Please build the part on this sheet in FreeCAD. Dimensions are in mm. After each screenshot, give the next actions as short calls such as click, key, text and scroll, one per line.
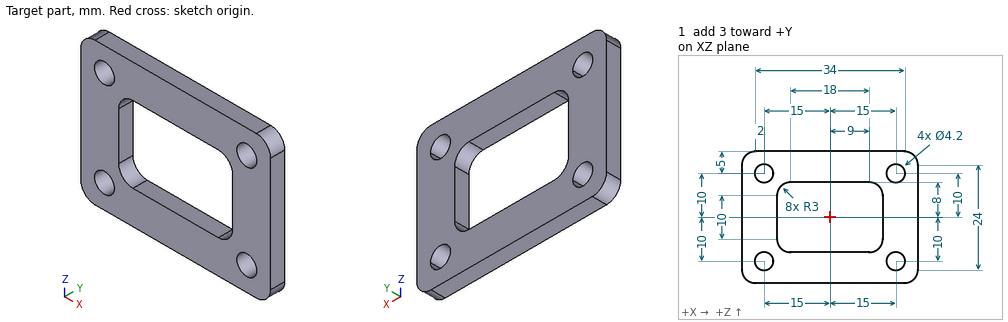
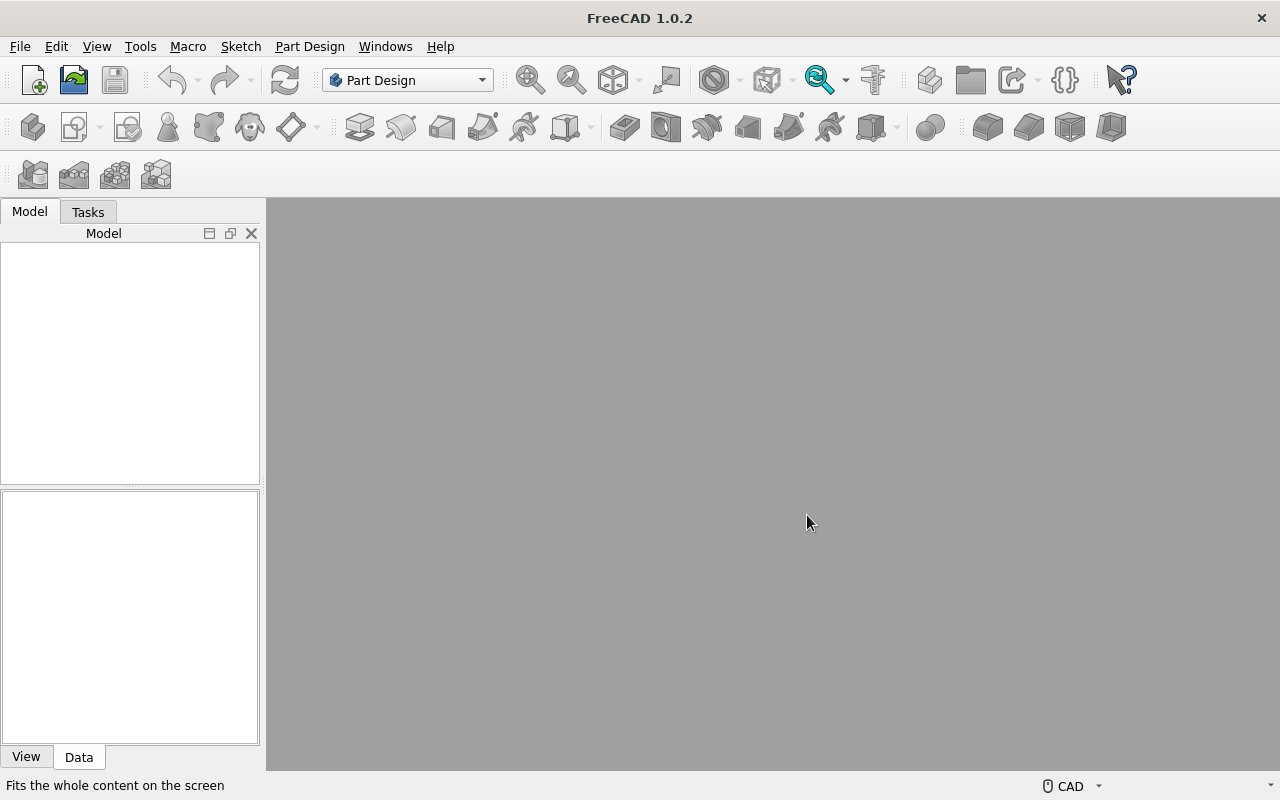
click(33, 80)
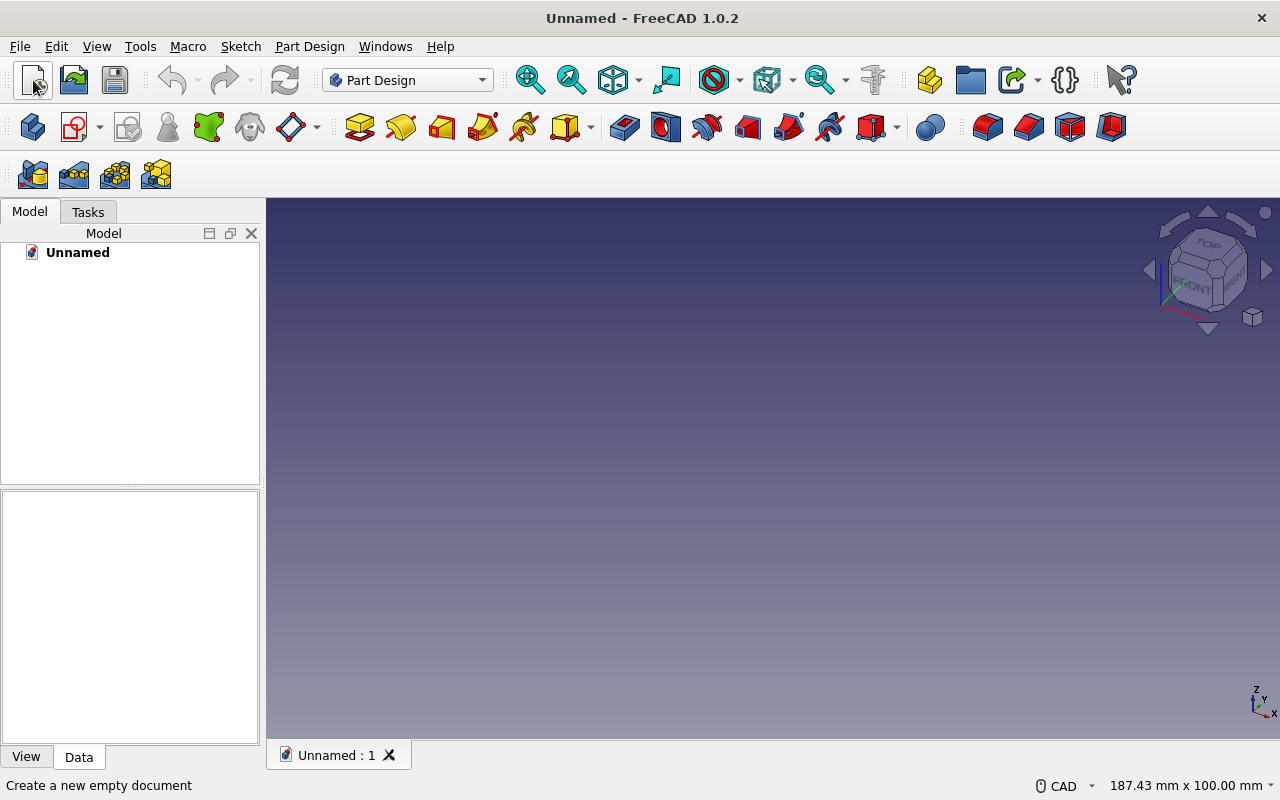
click(74, 128)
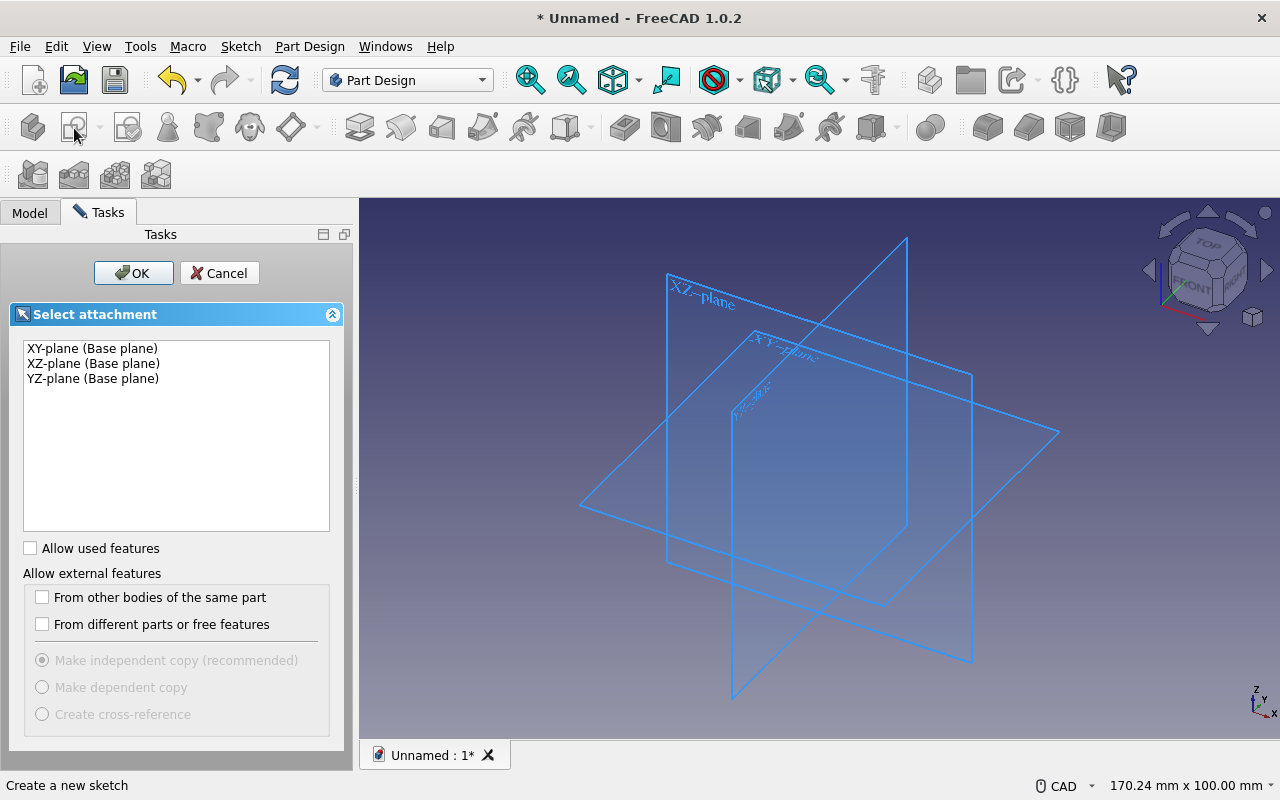
click(84, 364)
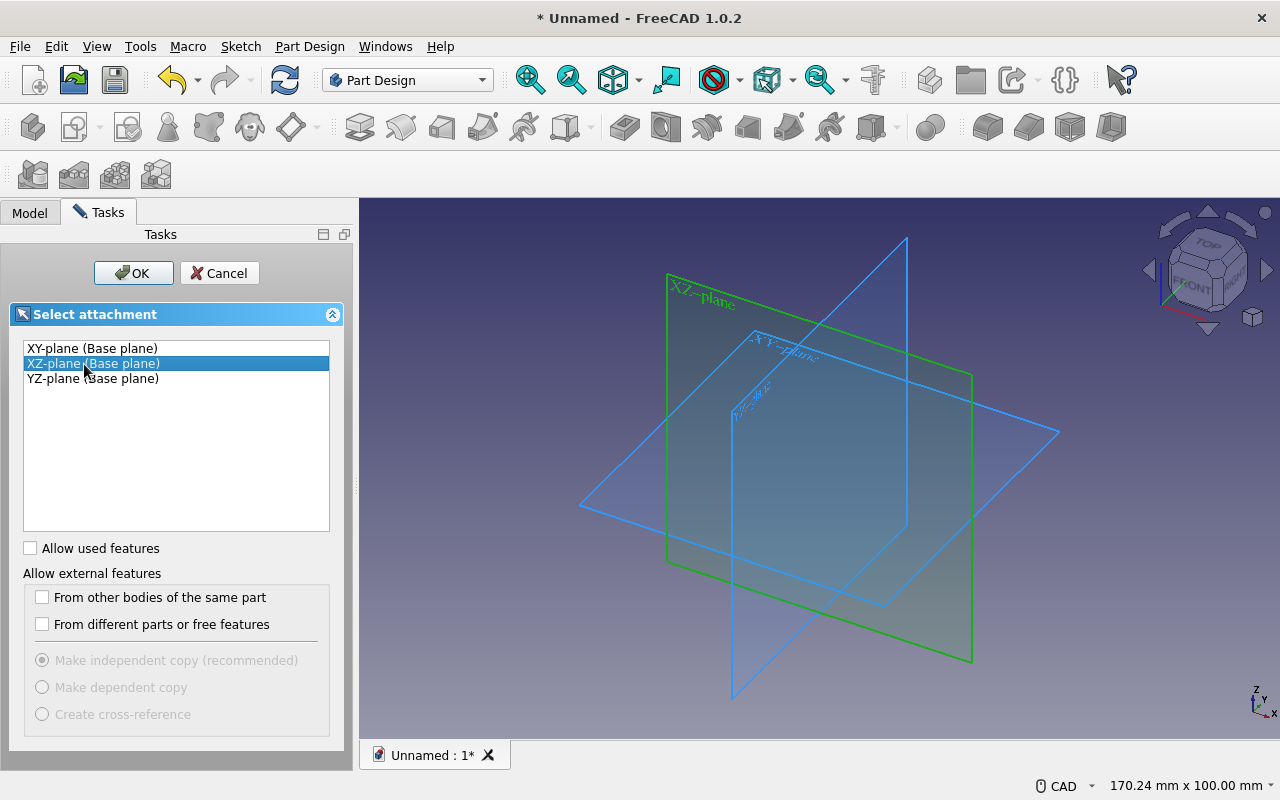
click(134, 273)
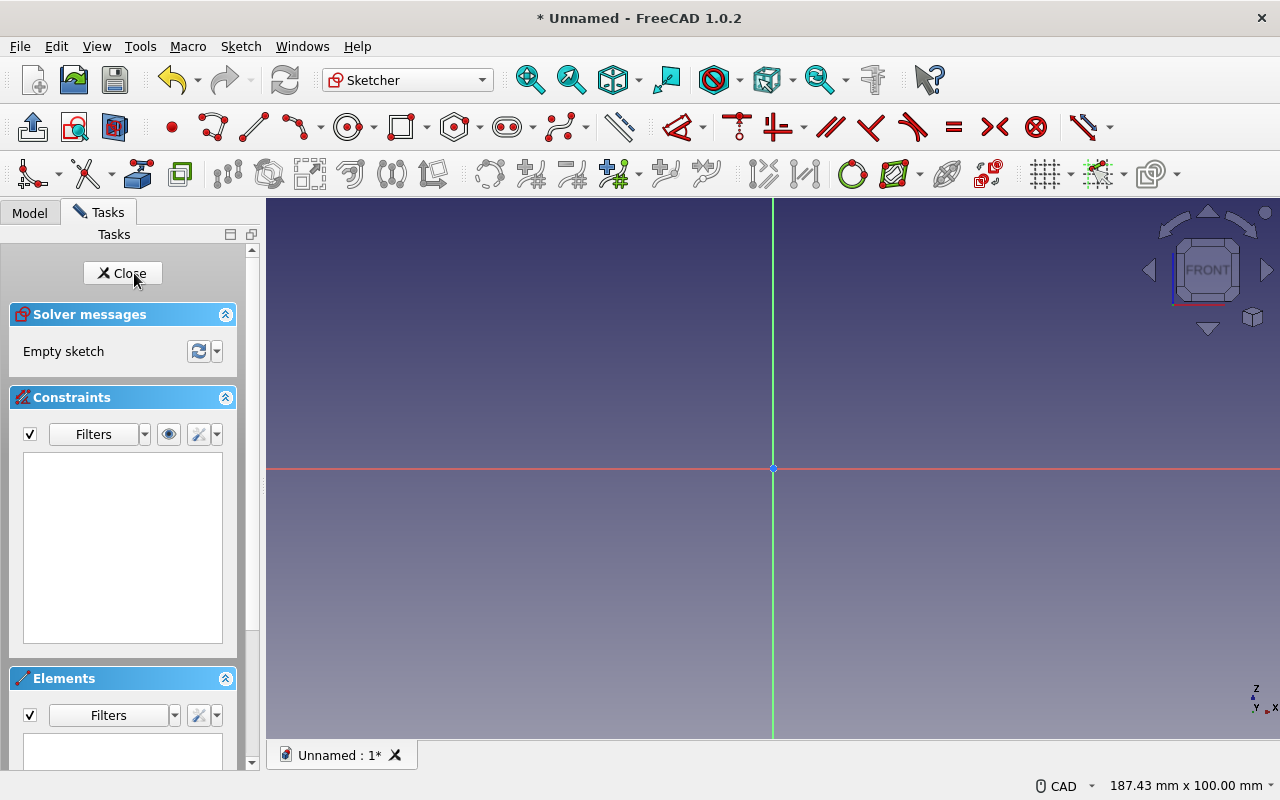
scroll(829, 469, up, 4)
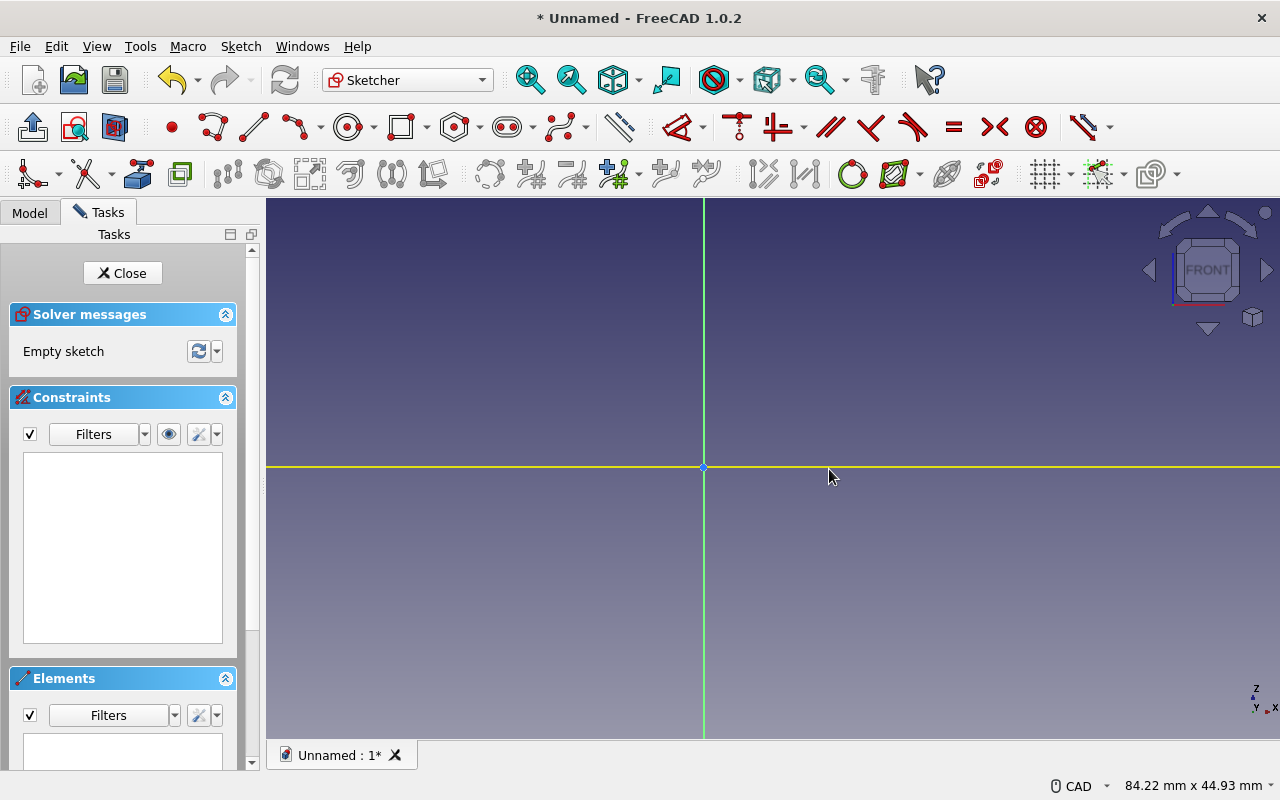
key(g)
key(l)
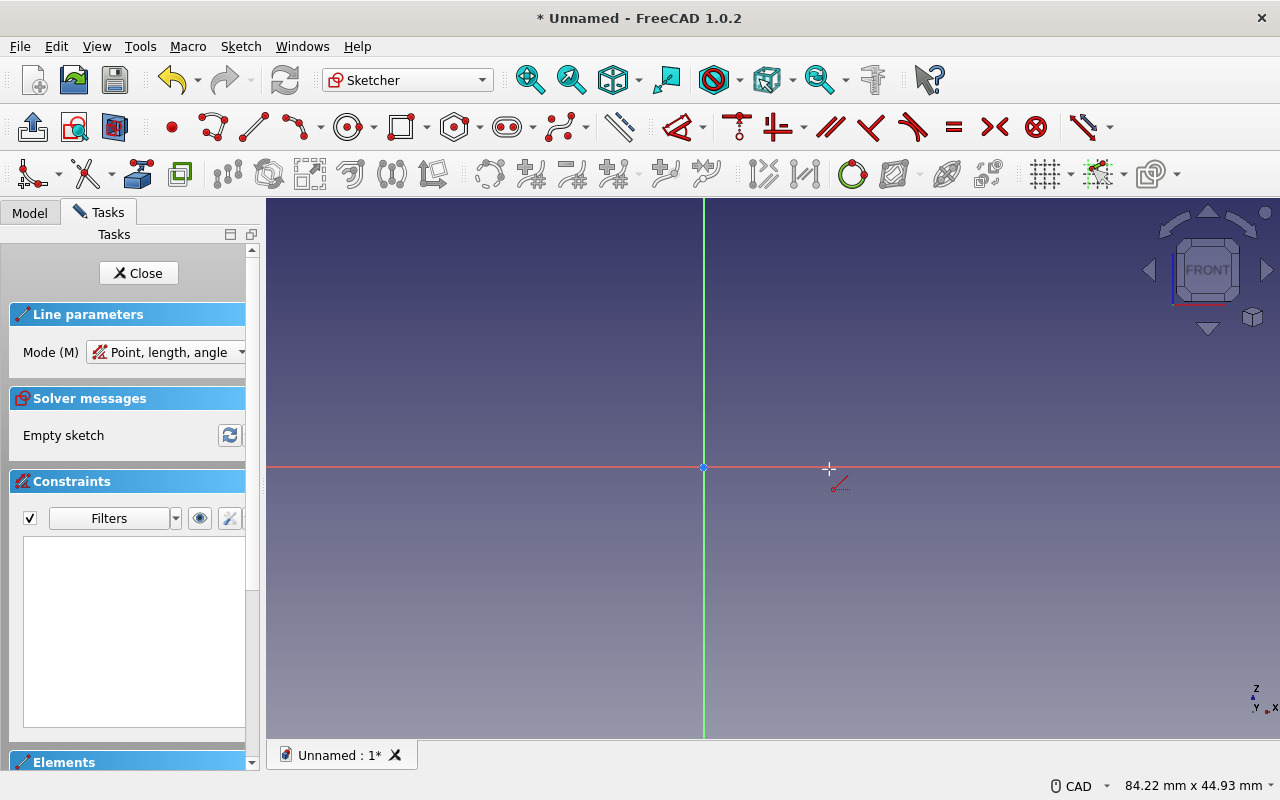
click(499, 287)
click(908, 287)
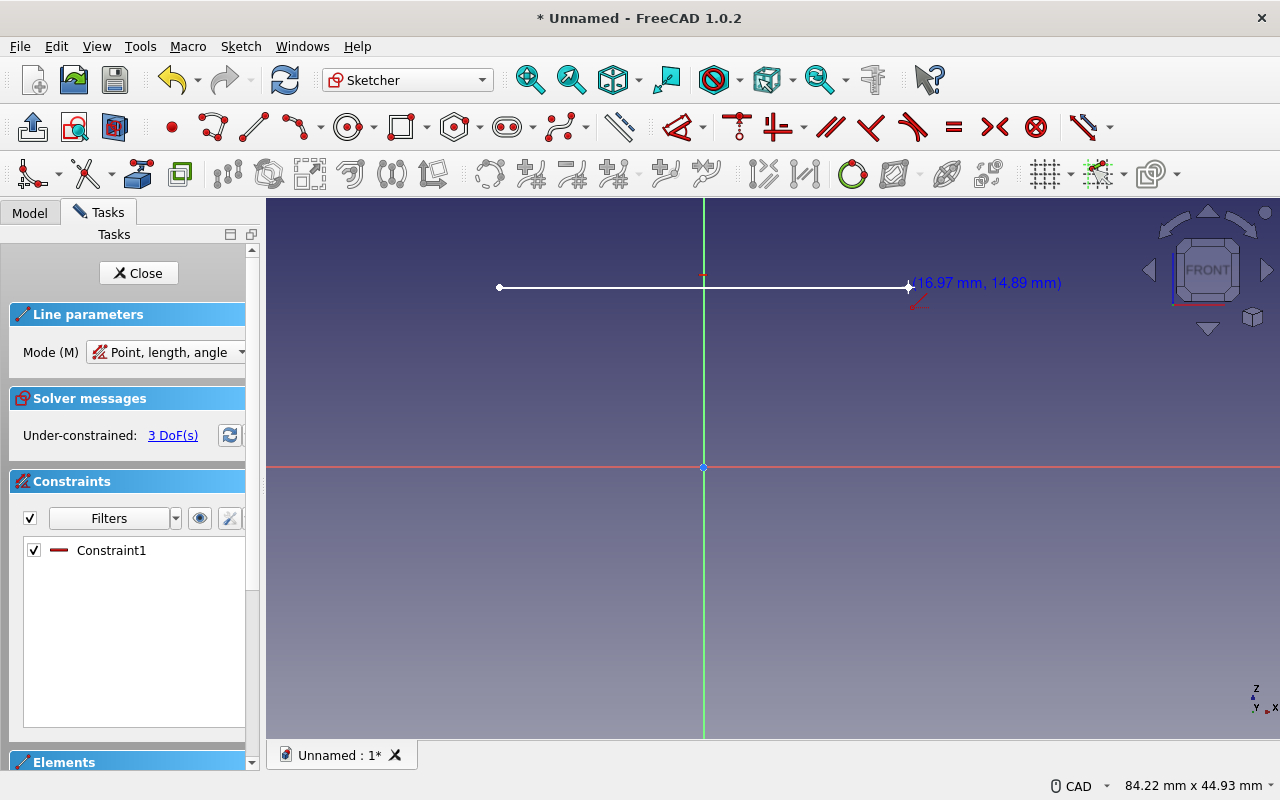
click(944, 323)
click(944, 612)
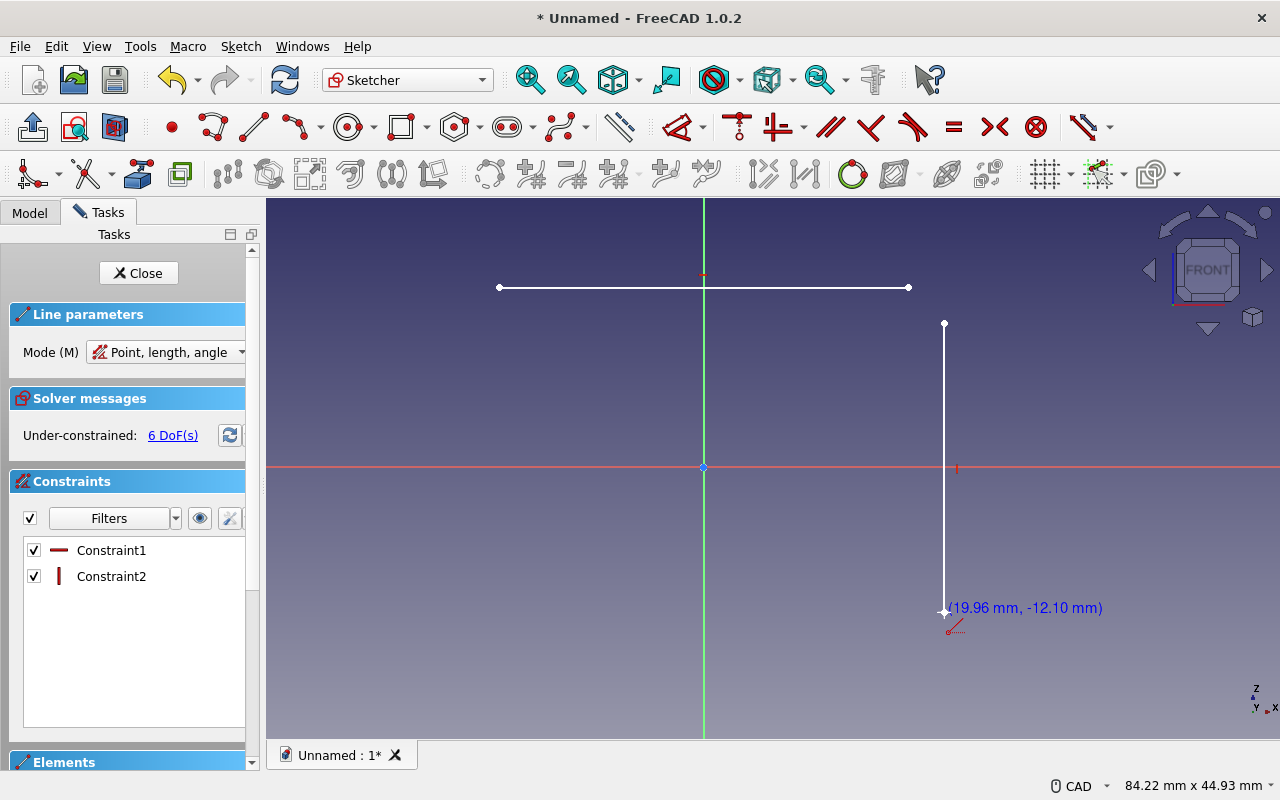
click(908, 648)
click(499, 648)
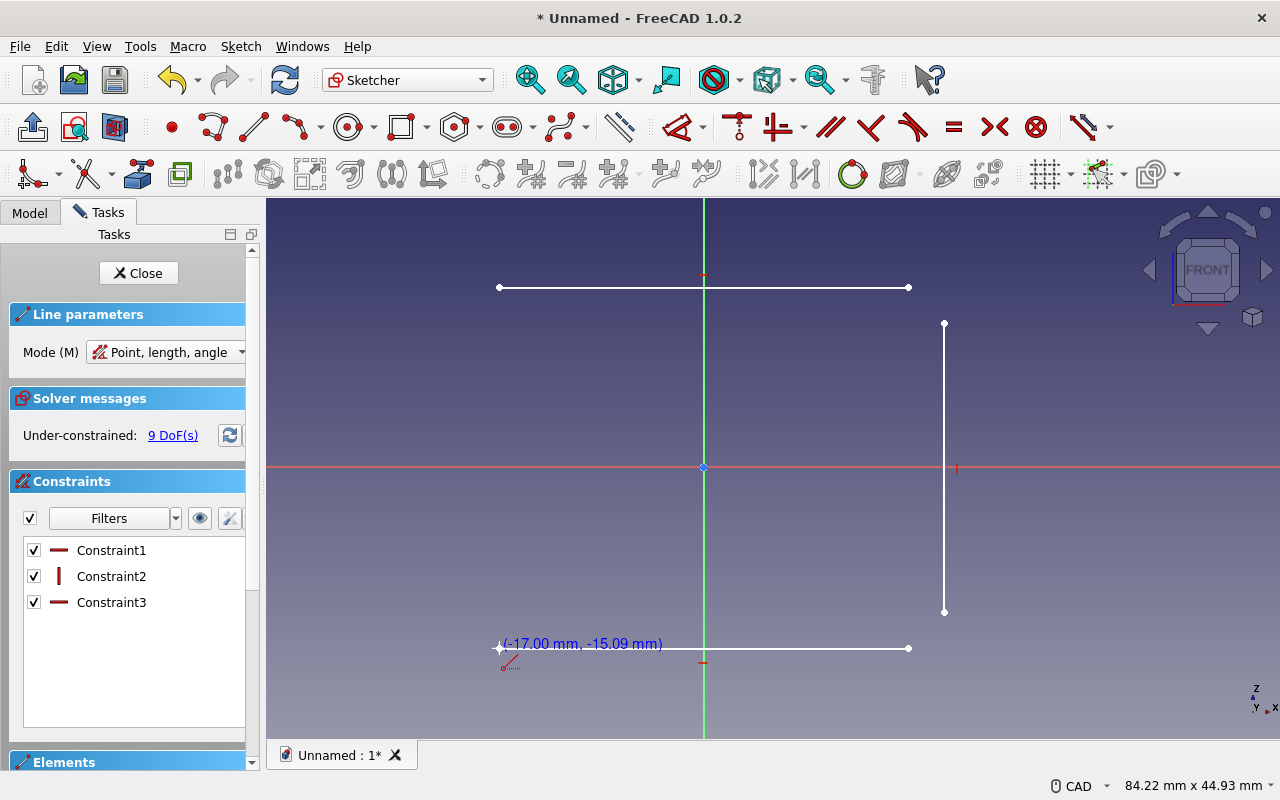
click(463, 612)
click(463, 323)